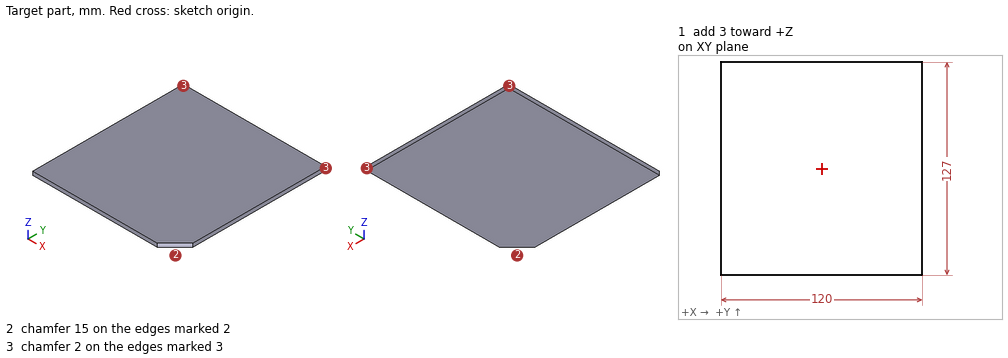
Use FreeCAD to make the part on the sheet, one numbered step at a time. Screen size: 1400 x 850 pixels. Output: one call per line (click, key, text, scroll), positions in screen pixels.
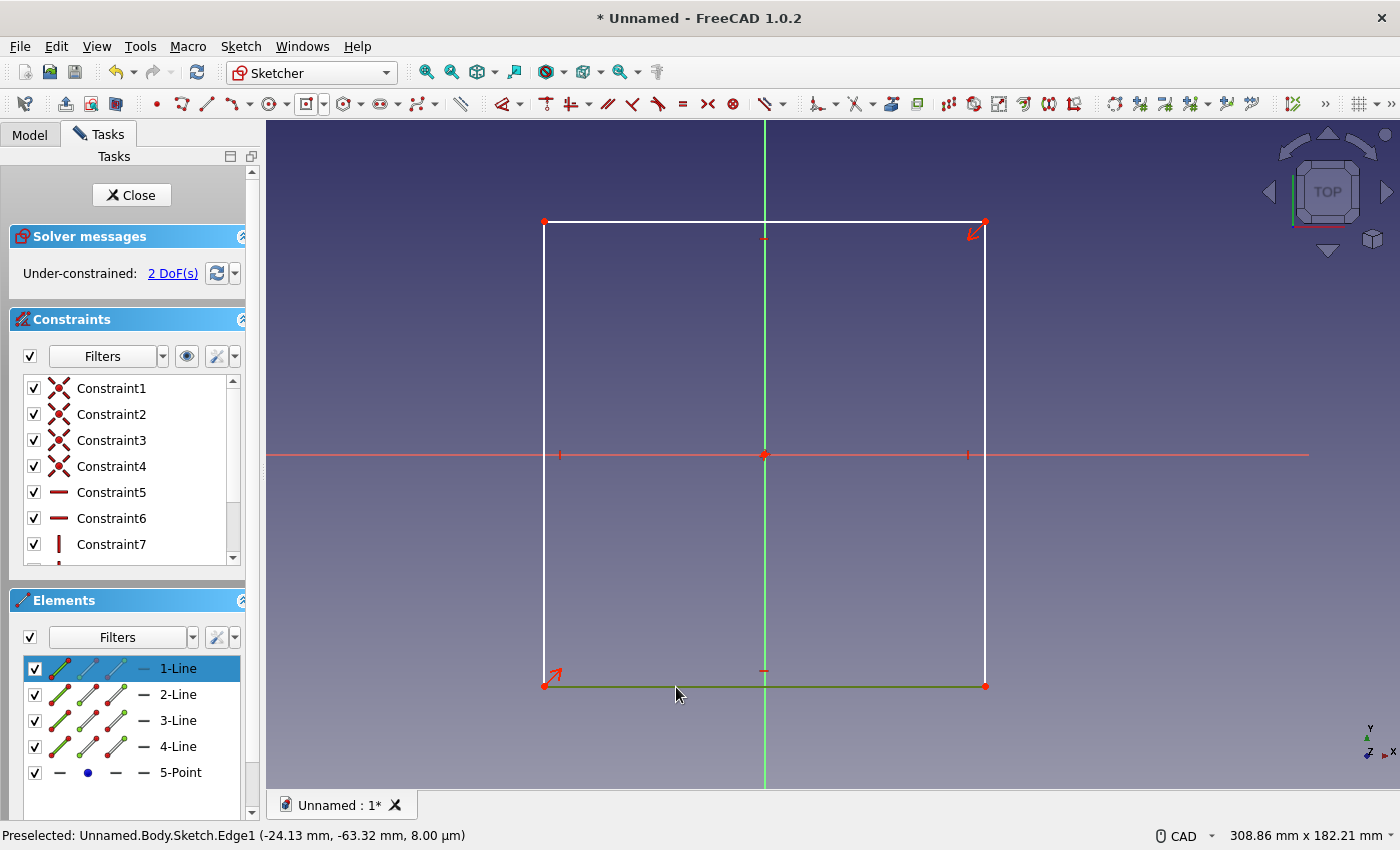
key(l)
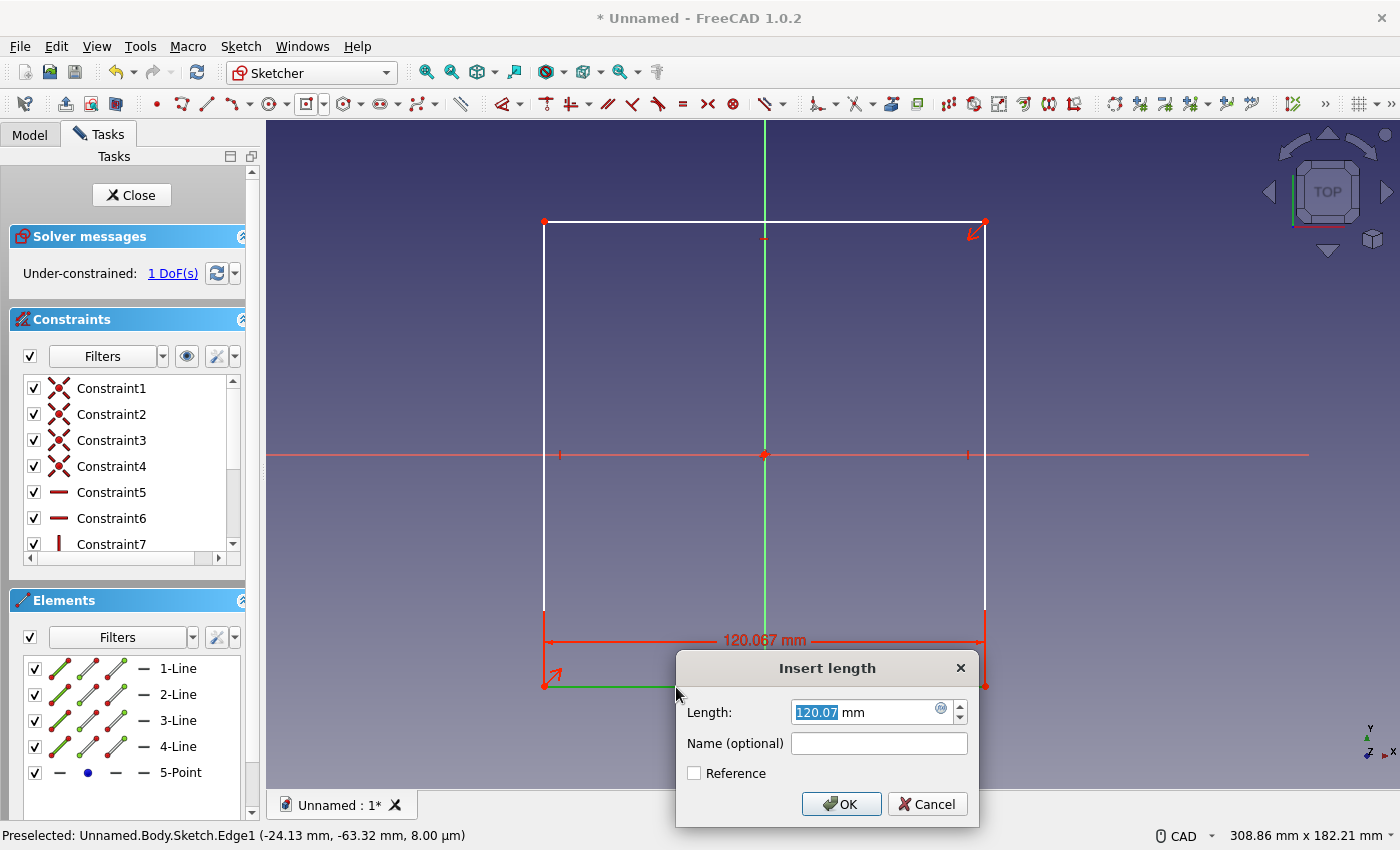
text(120)
key(Return)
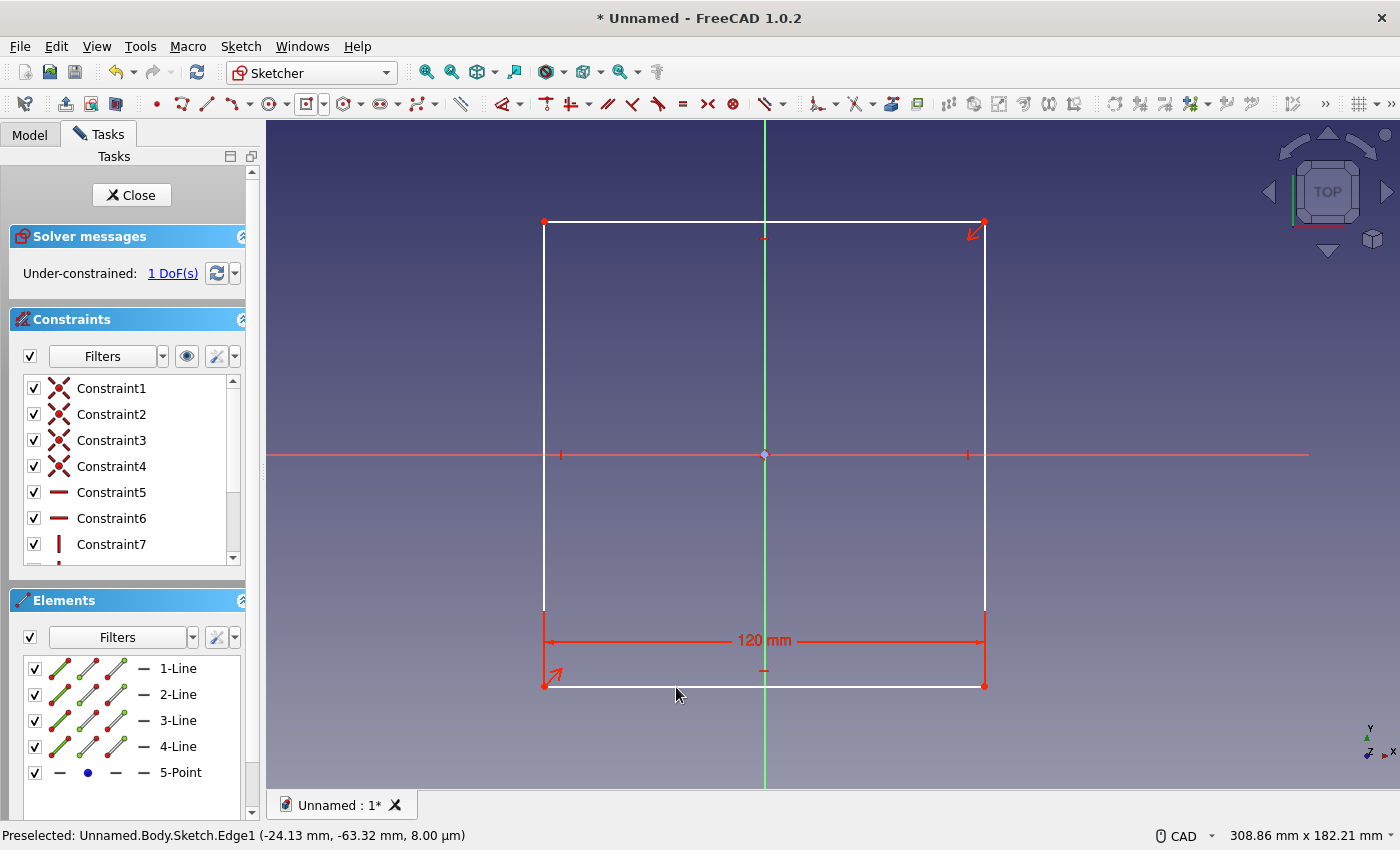
click(985, 548)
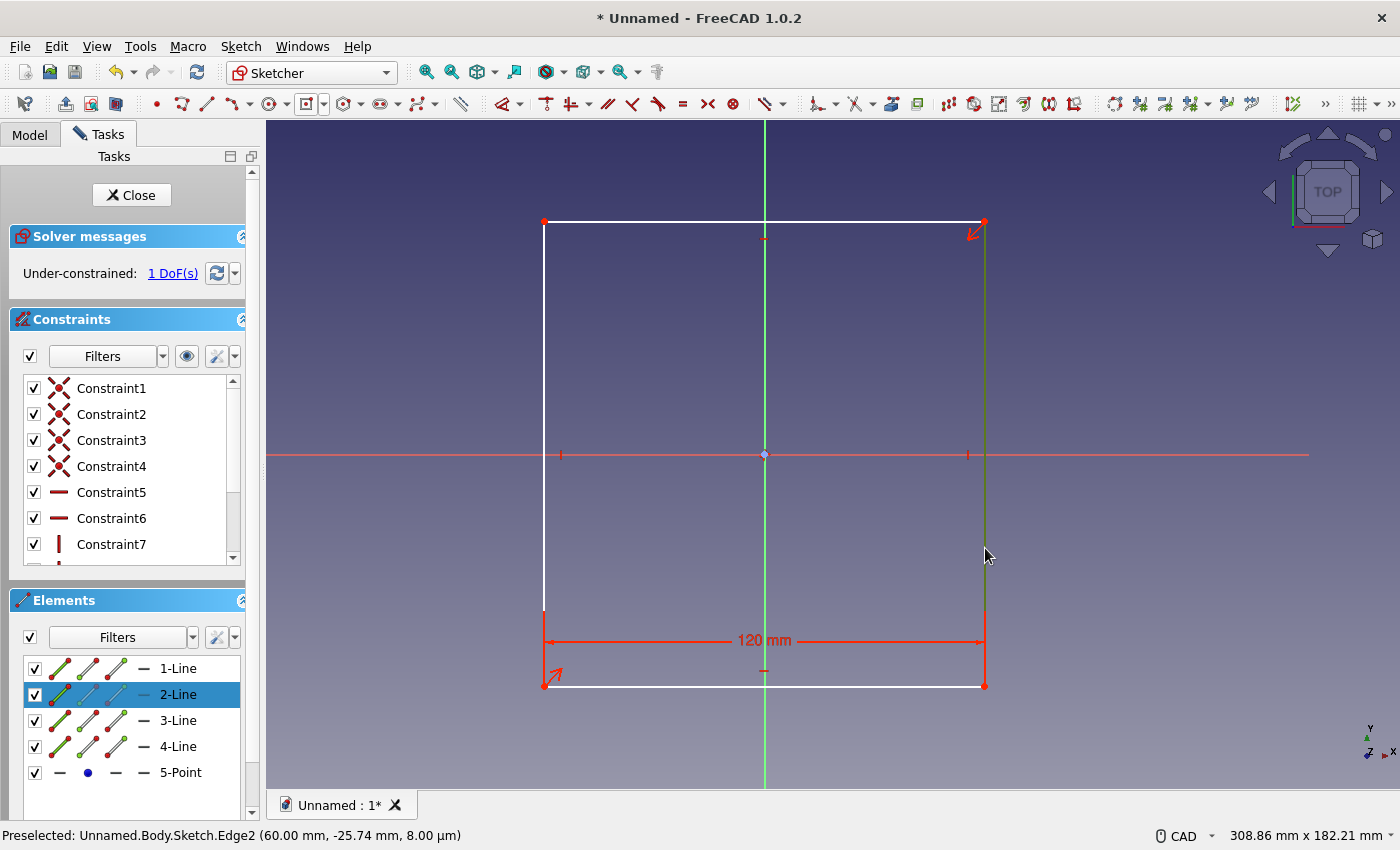
key(i)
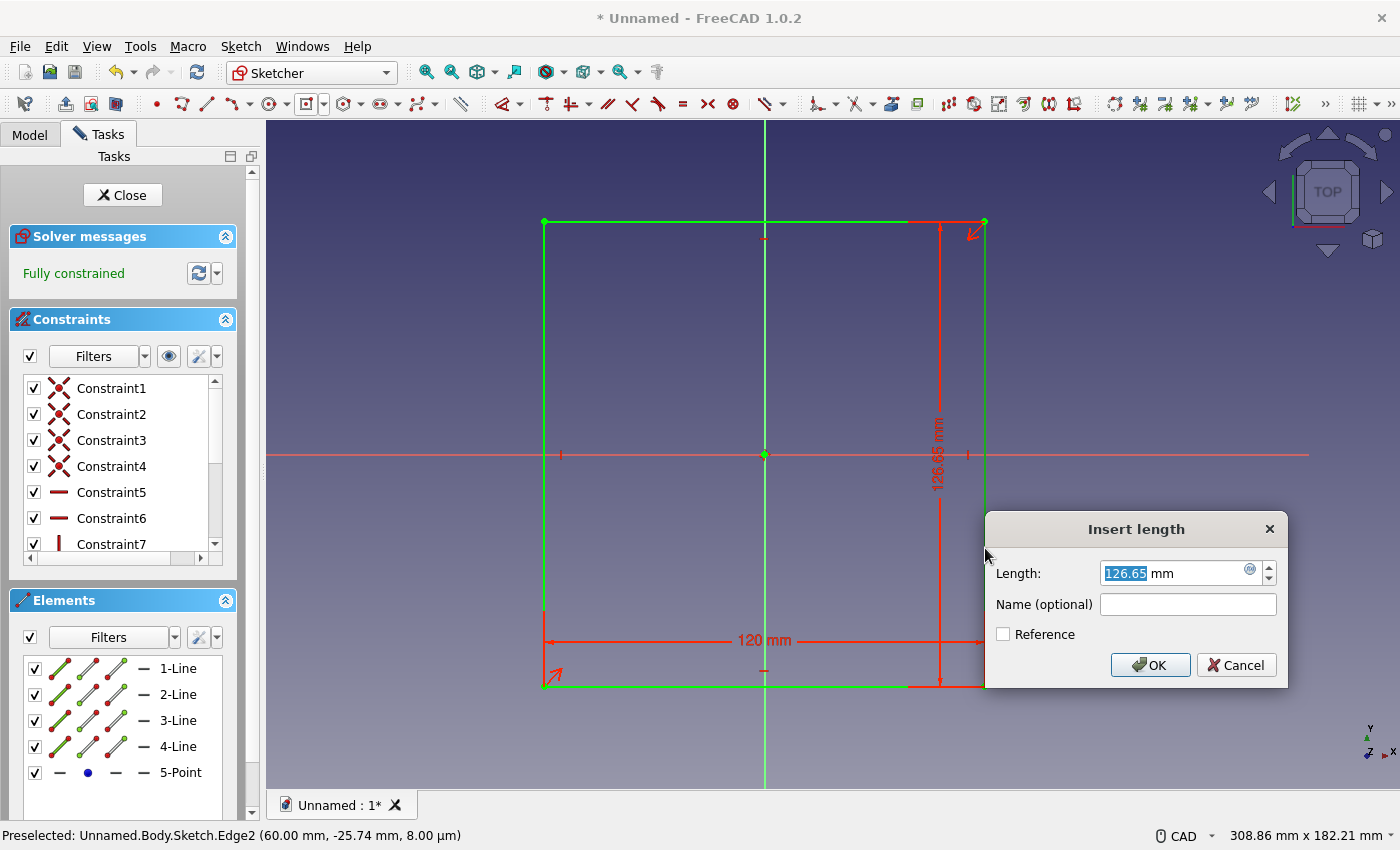
text(127)
key(Return)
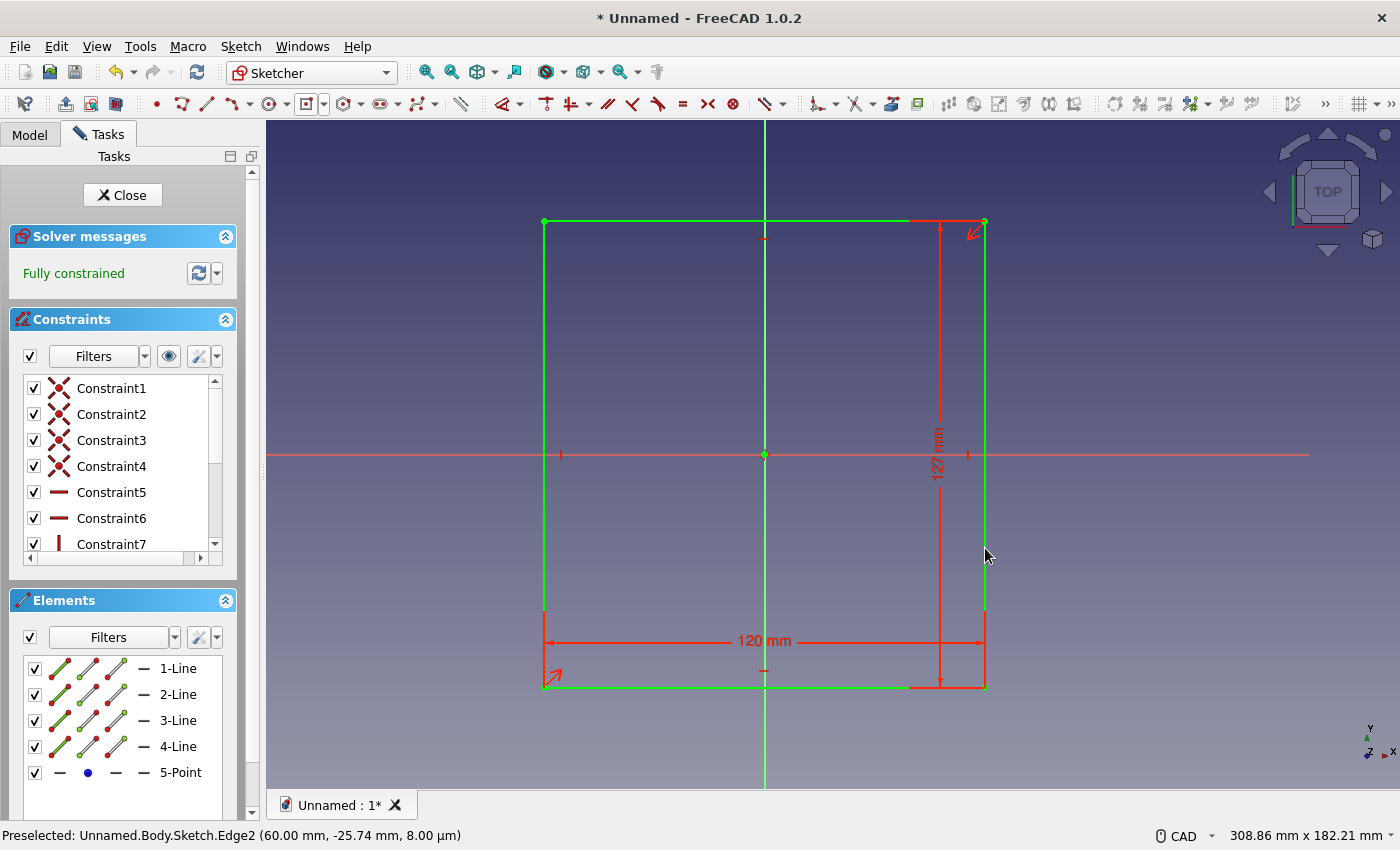
click(123, 195)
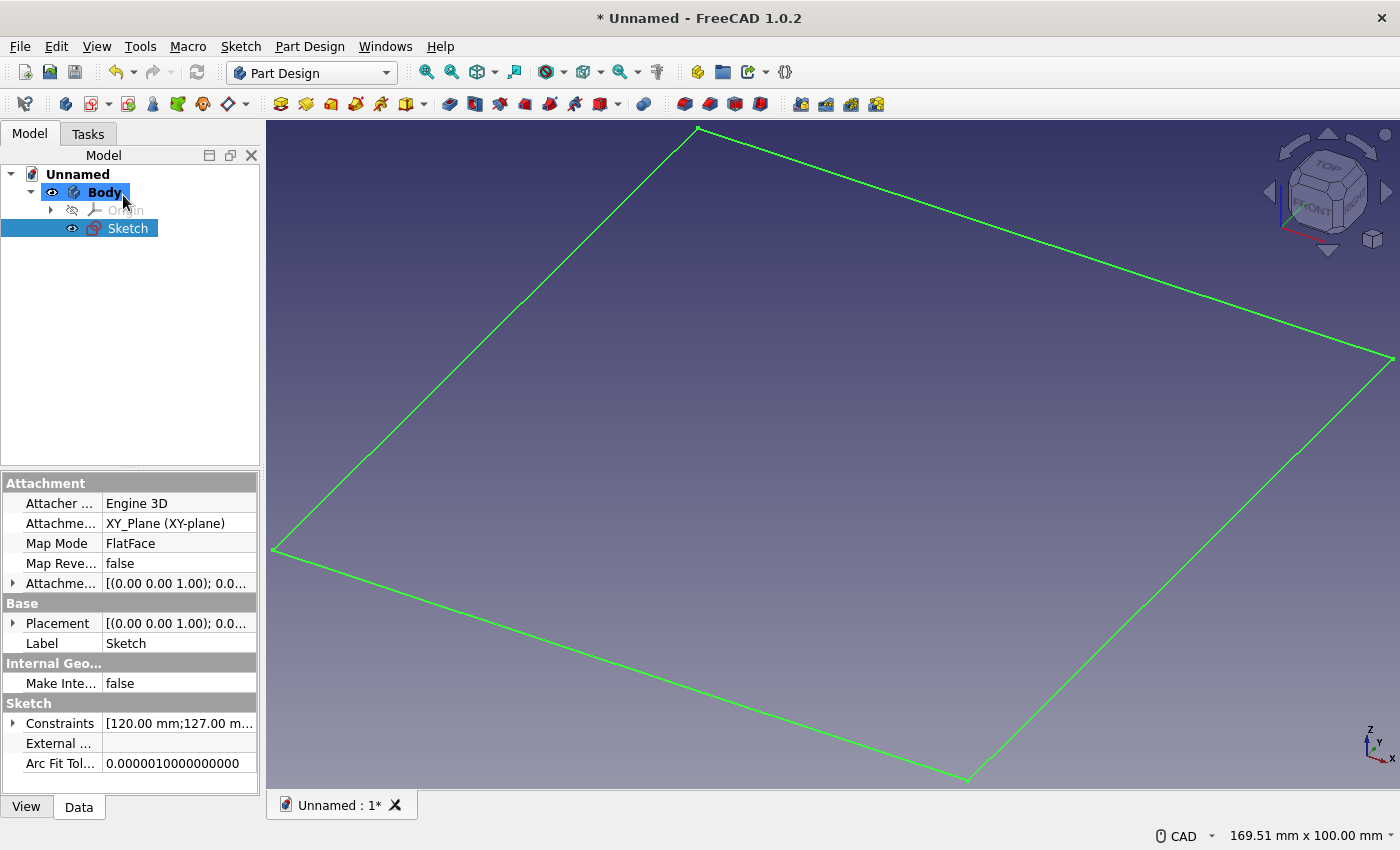
click(281, 104)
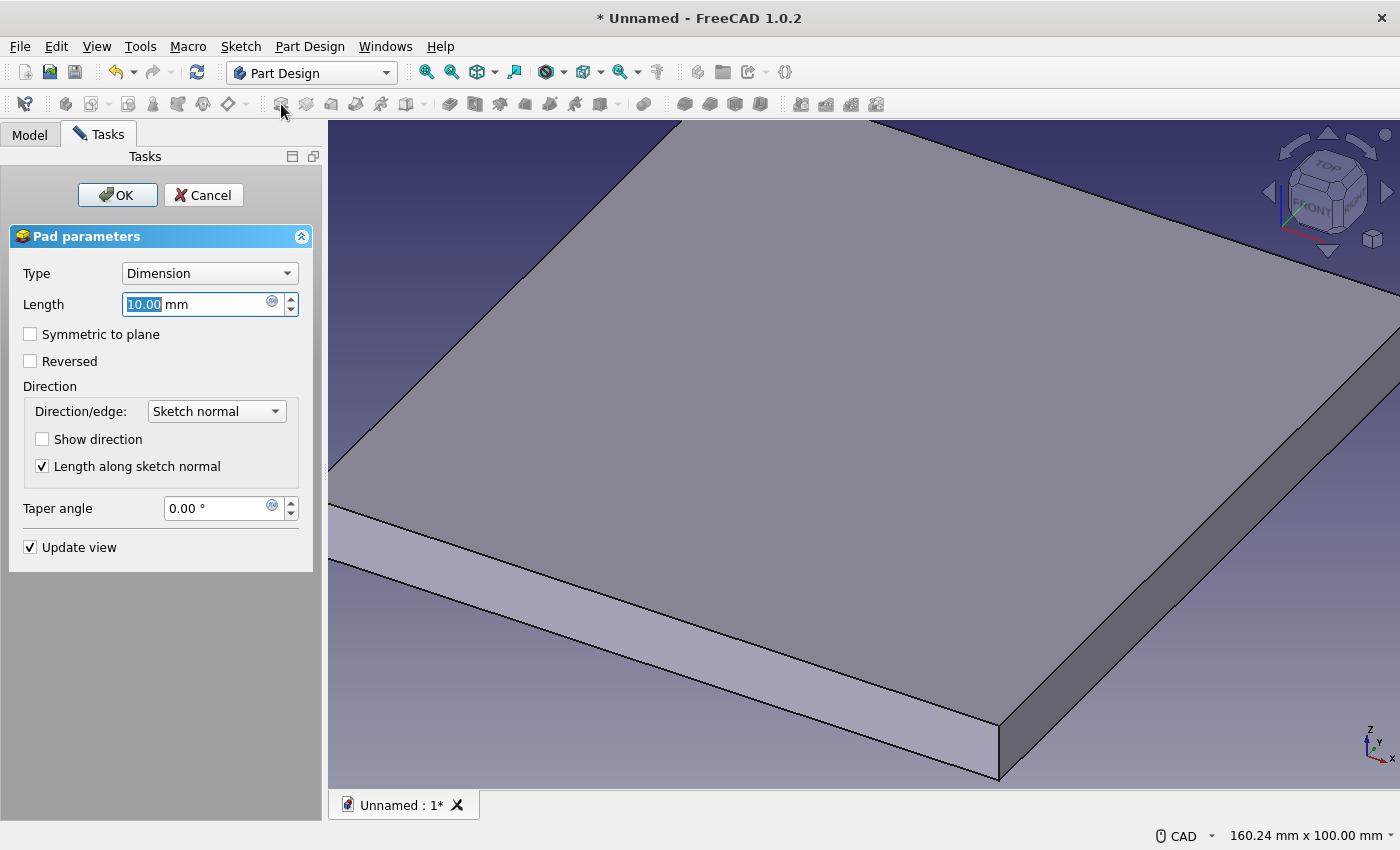
text(3)
key(Tab)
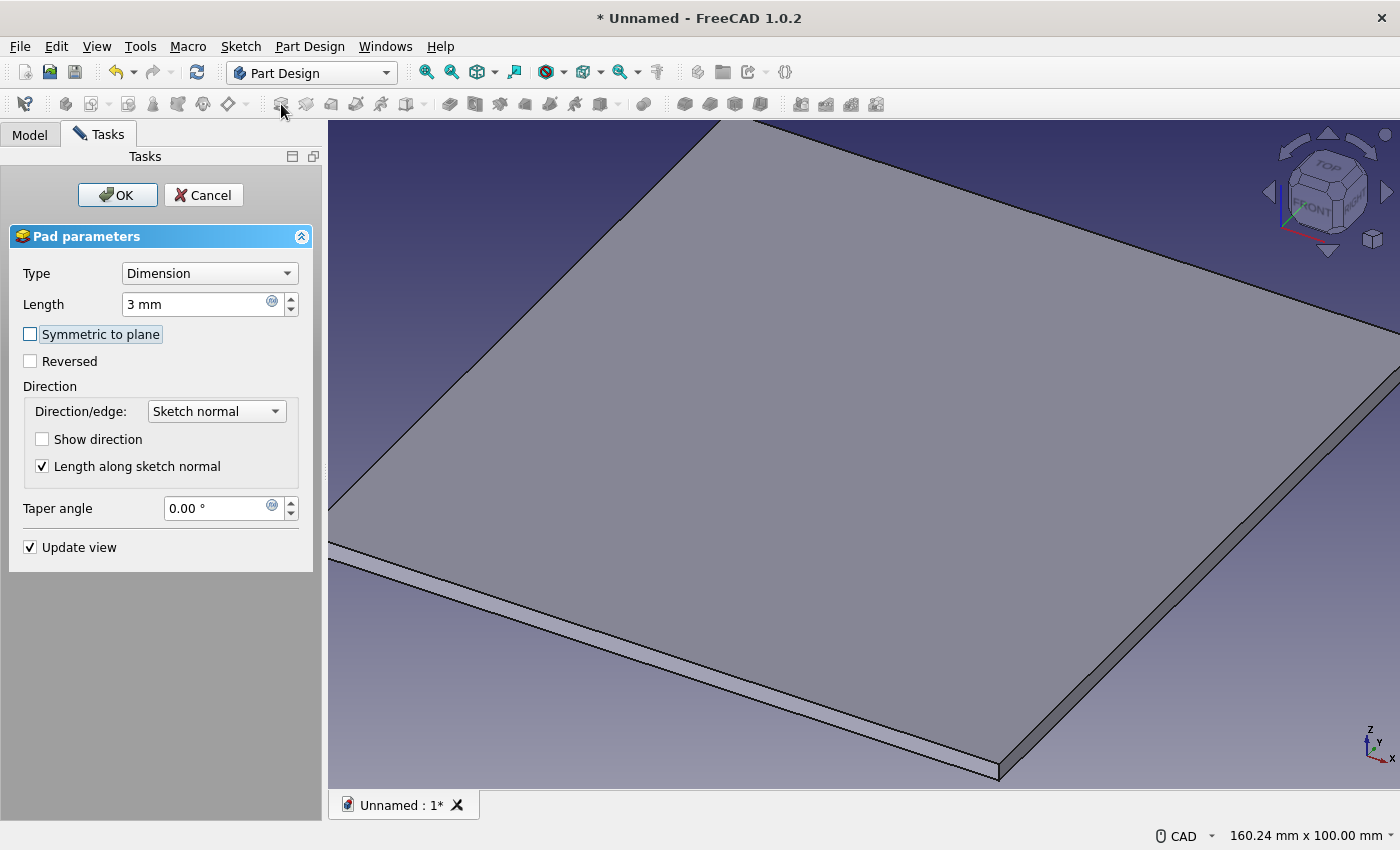
click(118, 195)